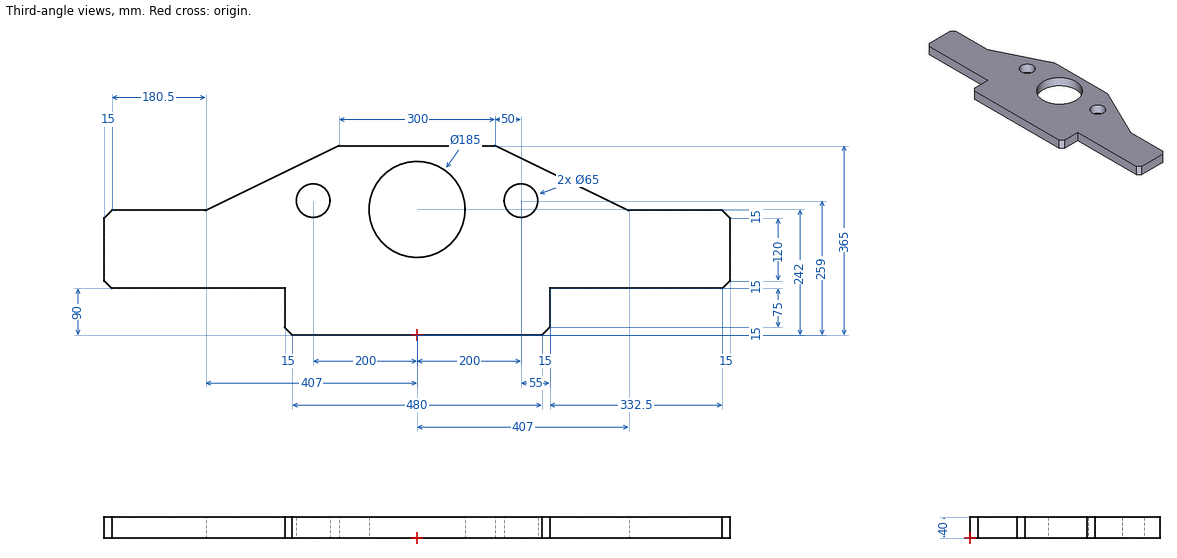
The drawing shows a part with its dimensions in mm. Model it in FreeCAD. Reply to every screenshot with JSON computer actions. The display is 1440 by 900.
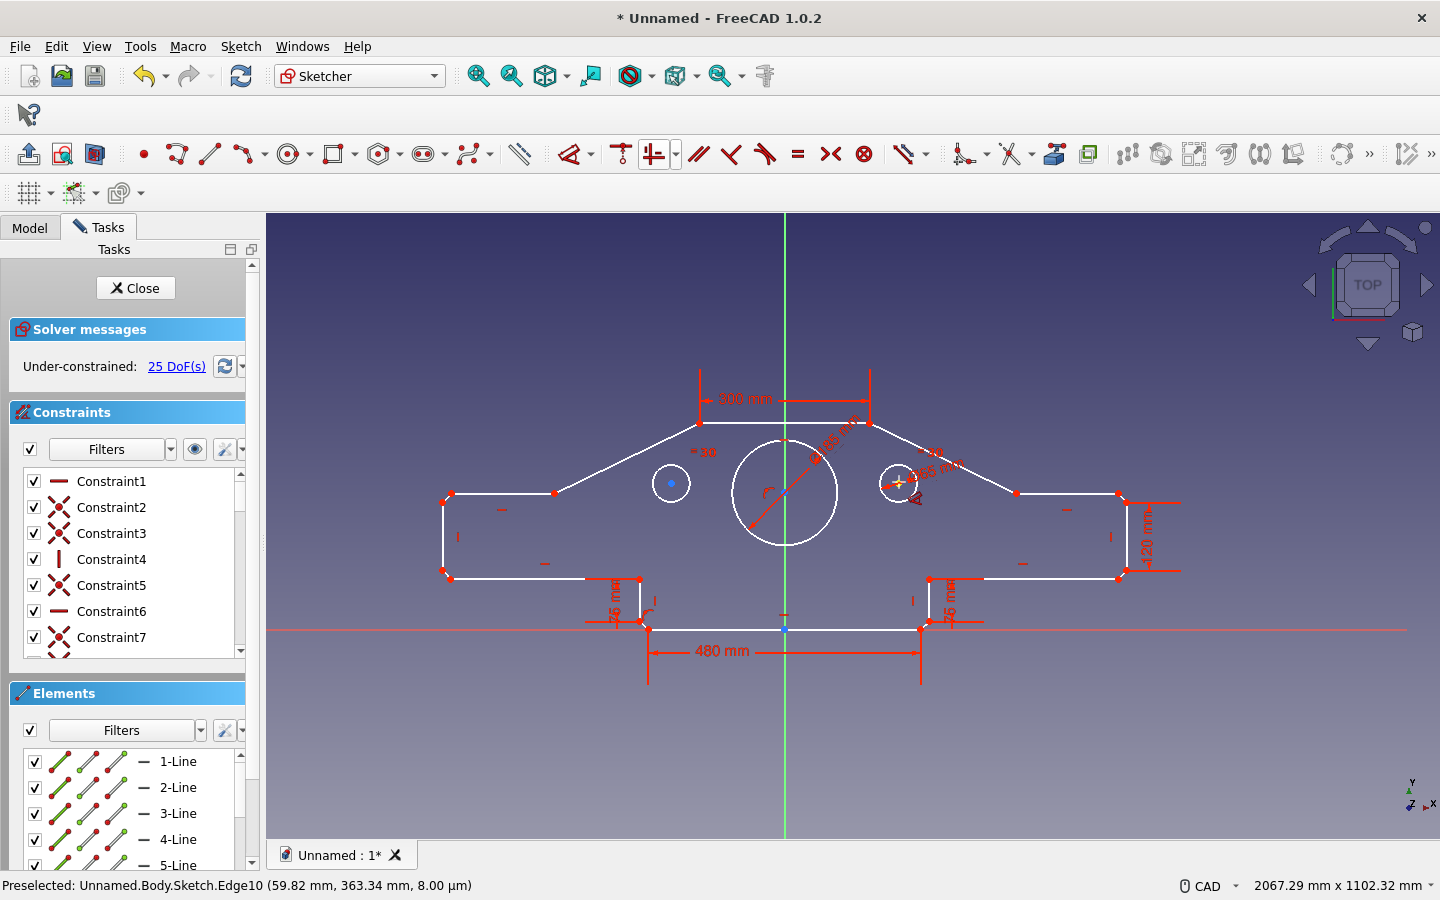
{"action": "left_click", "coordinate": [443, 523]}
{"action": "left_click", "coordinate": [409, 537]}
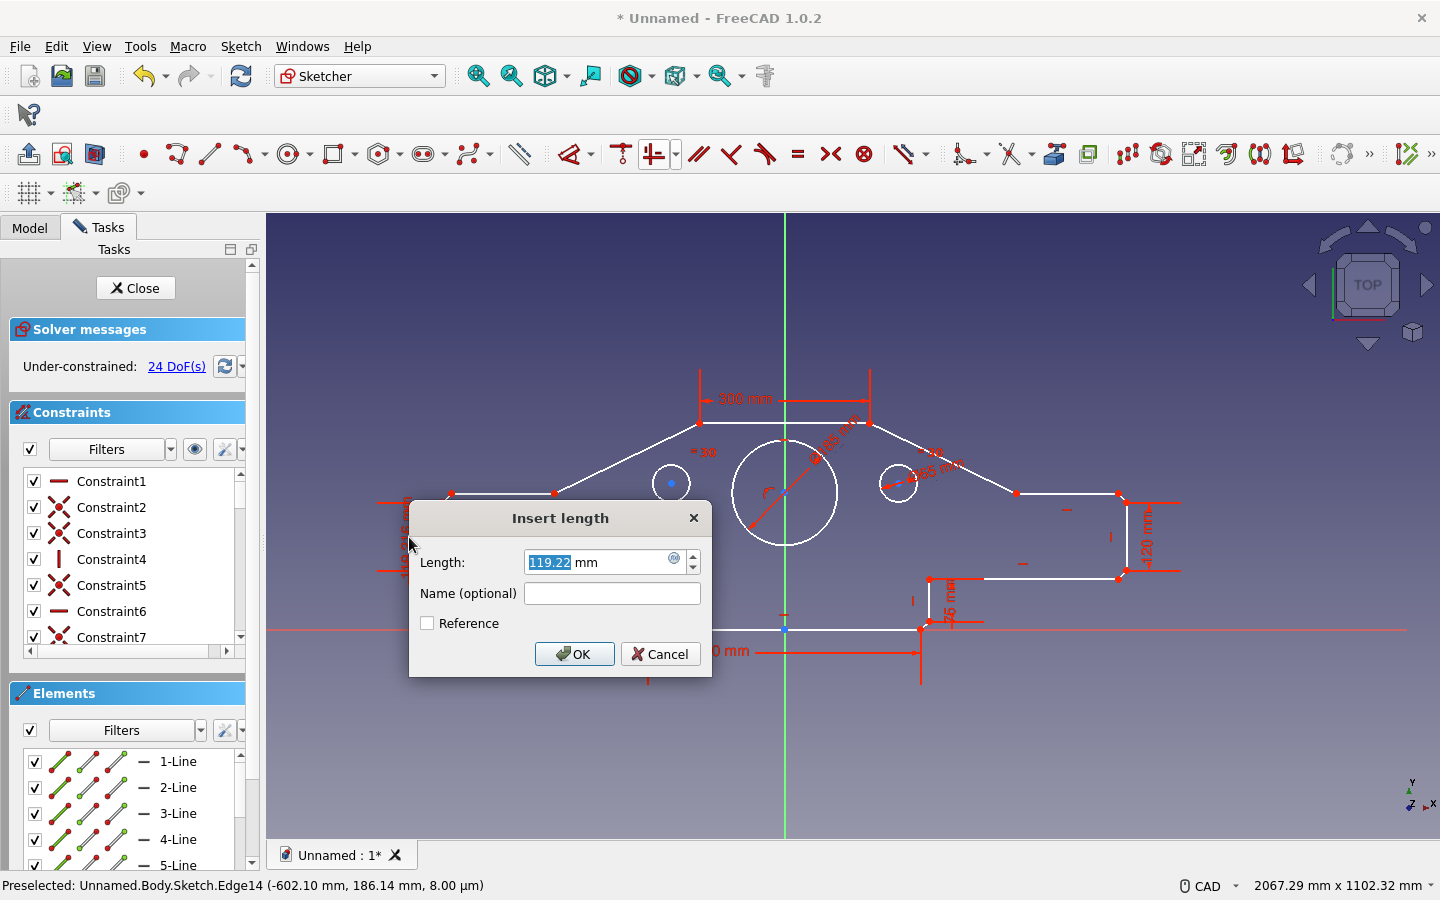
{"action": "type", "text": "120"}
{"action": "key", "text": "Return"}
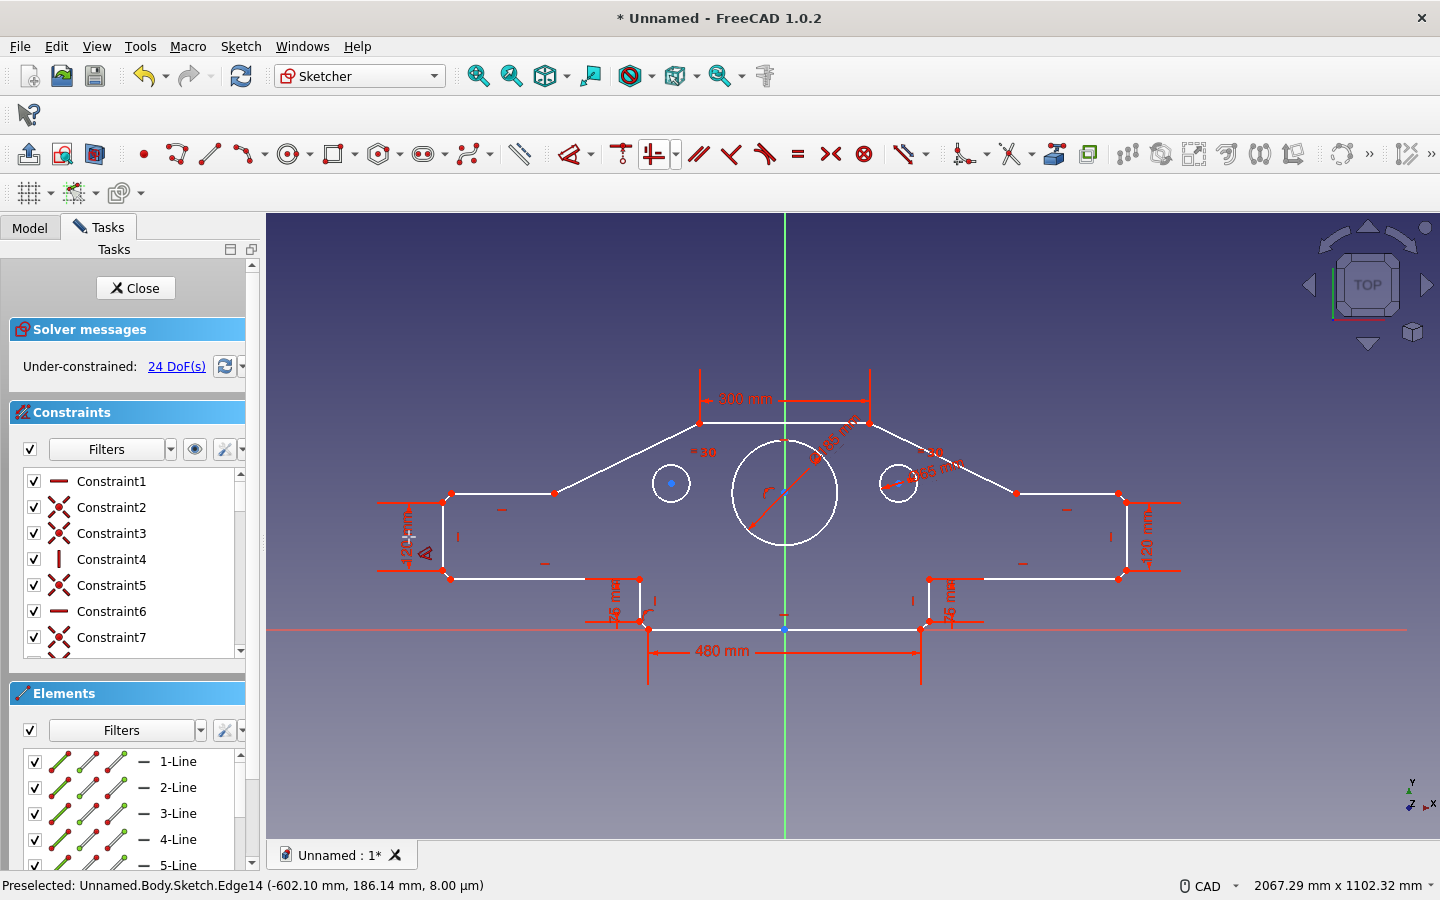
{"action": "scroll", "coordinate": [929, 622], "scroll_direction": "up", "scroll_amount": 8}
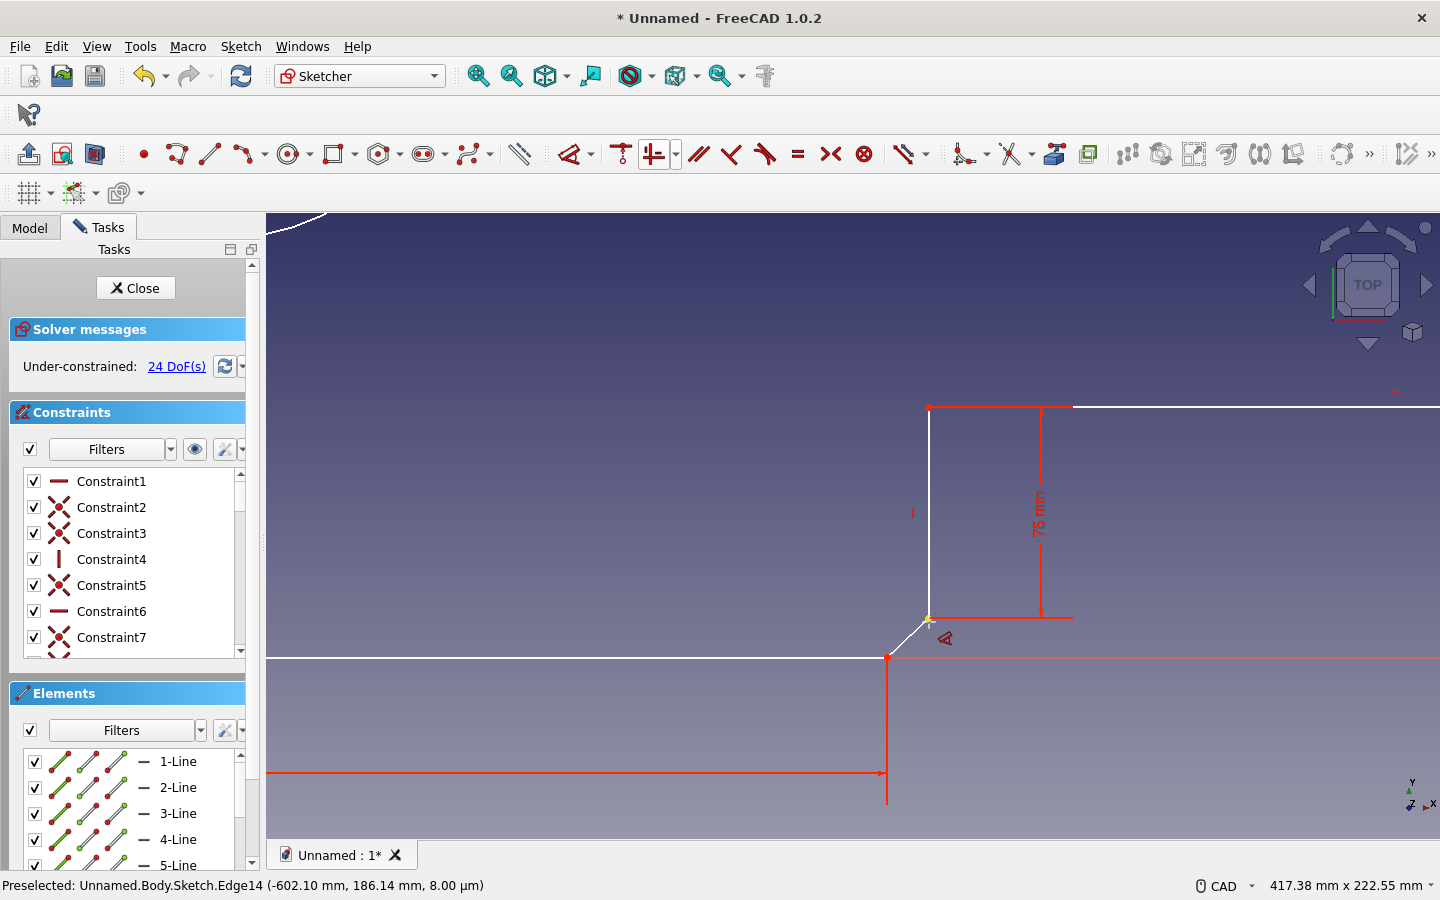
{"action": "left_click", "coordinate": [929, 618]}
{"action": "left_click", "coordinate": [963, 638]}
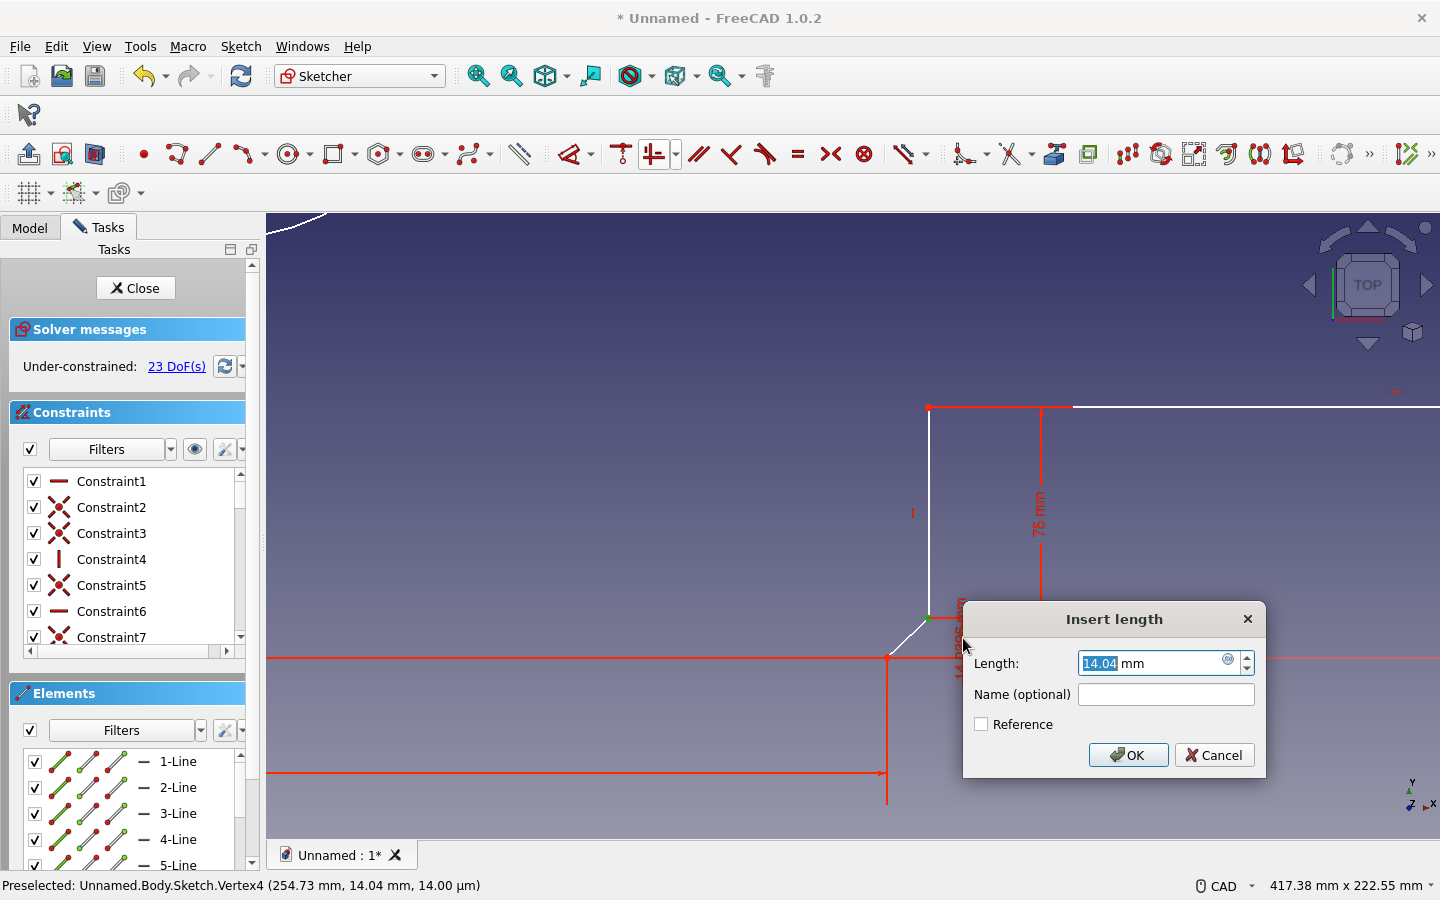
{"action": "type", "text": "15"}
{"action": "key", "text": "Return"}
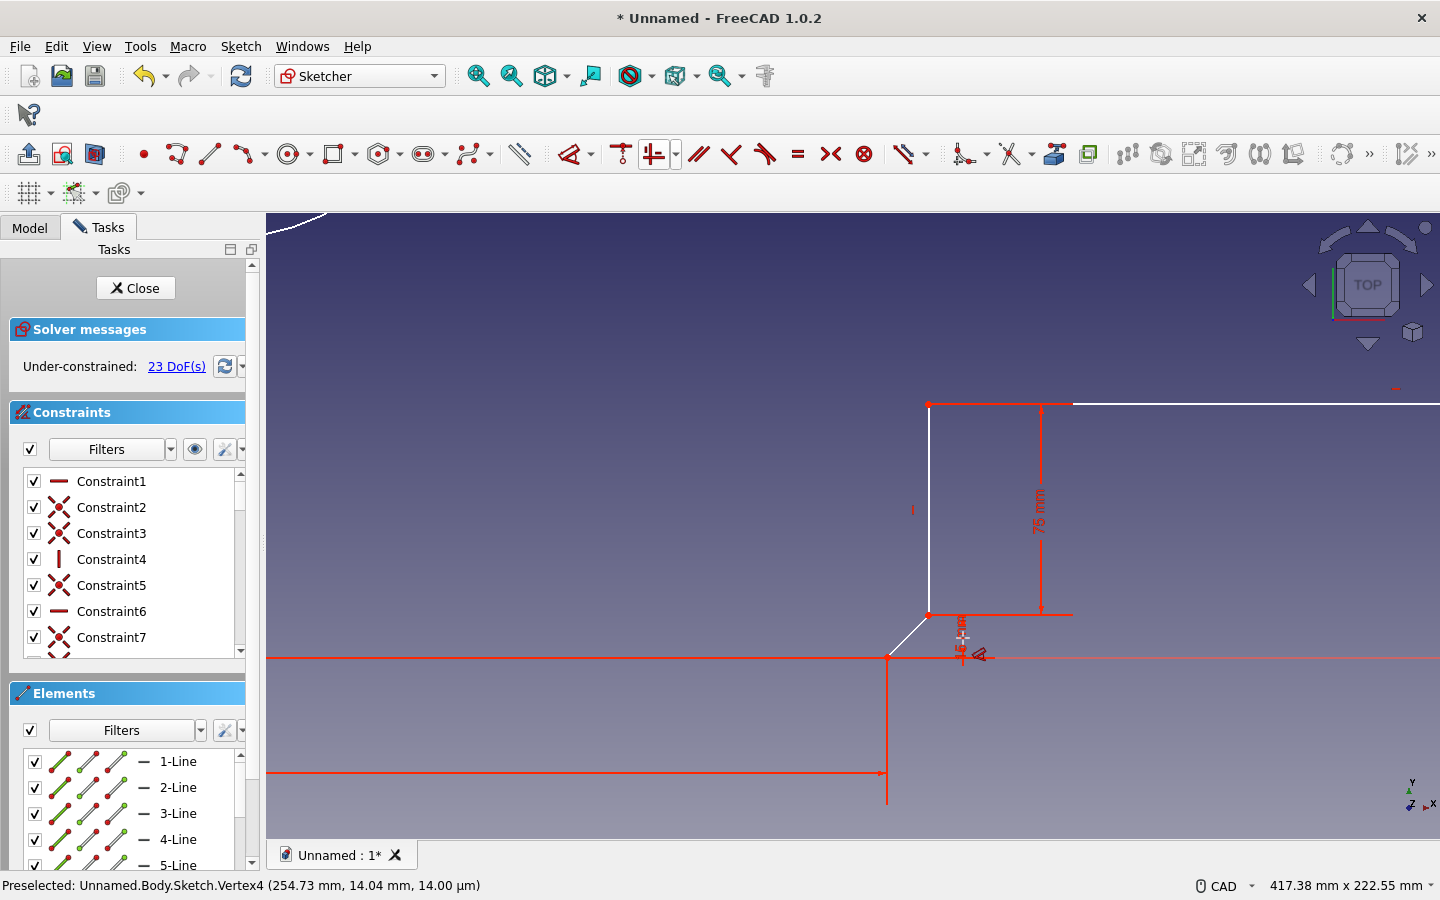
{"action": "scroll", "coordinate": [929, 623], "scroll_direction": "down", "scroll_amount": 8}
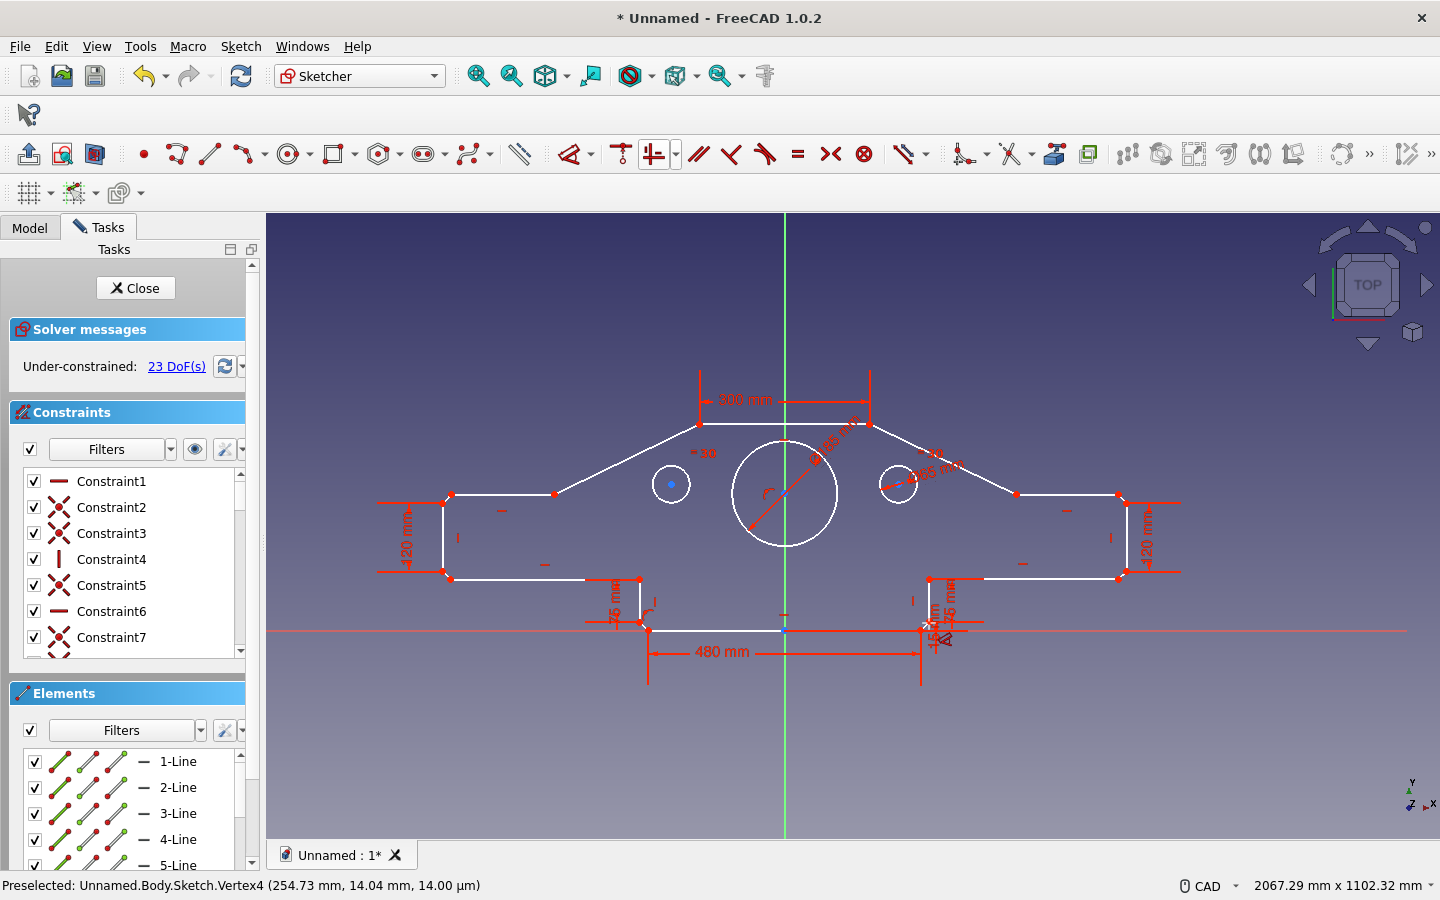
{"action": "left_click", "coordinate": [451, 580]}
{"action": "left_click", "coordinate": [417, 605]}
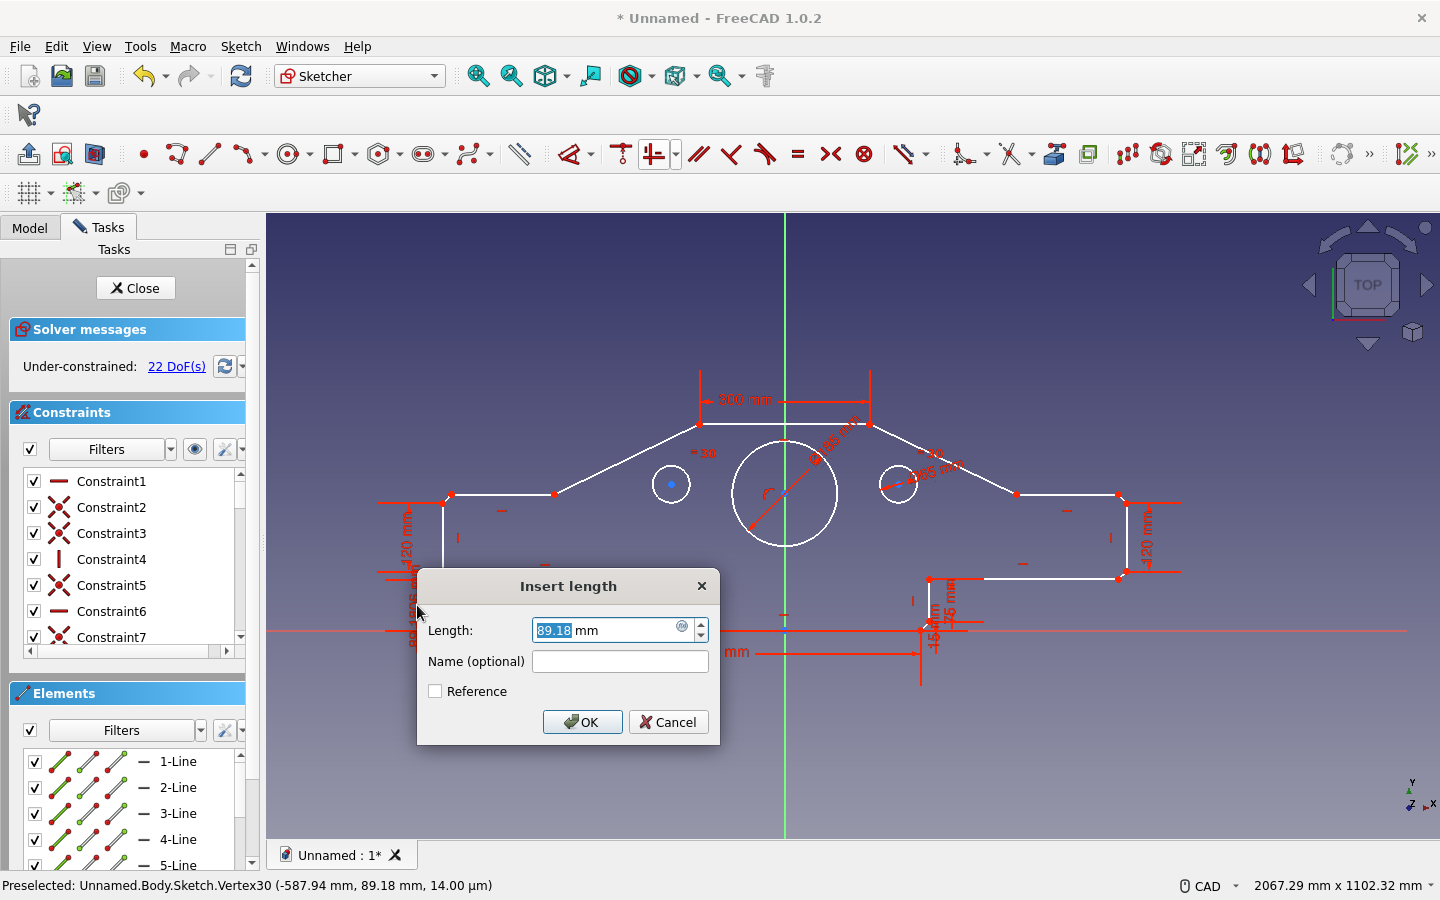
{"action": "type", "text": "90"}
{"action": "key", "text": "Return"}